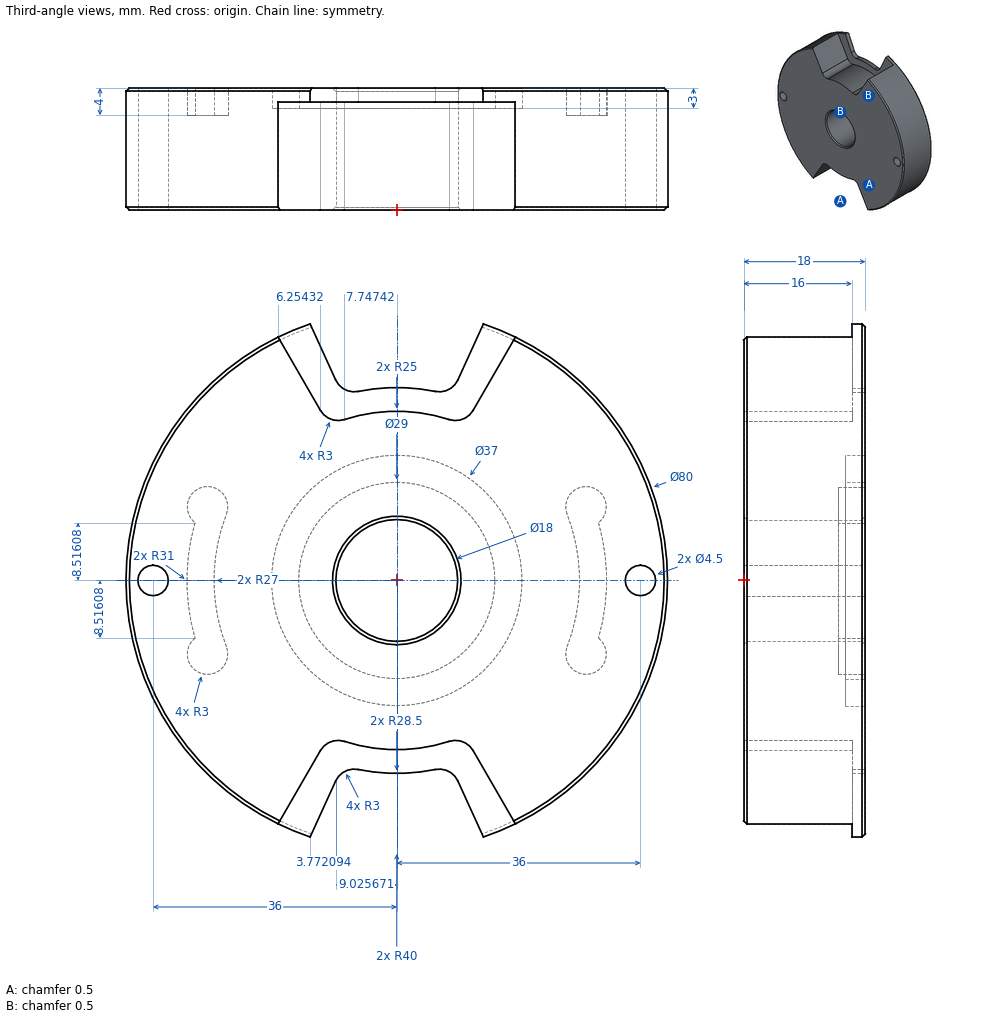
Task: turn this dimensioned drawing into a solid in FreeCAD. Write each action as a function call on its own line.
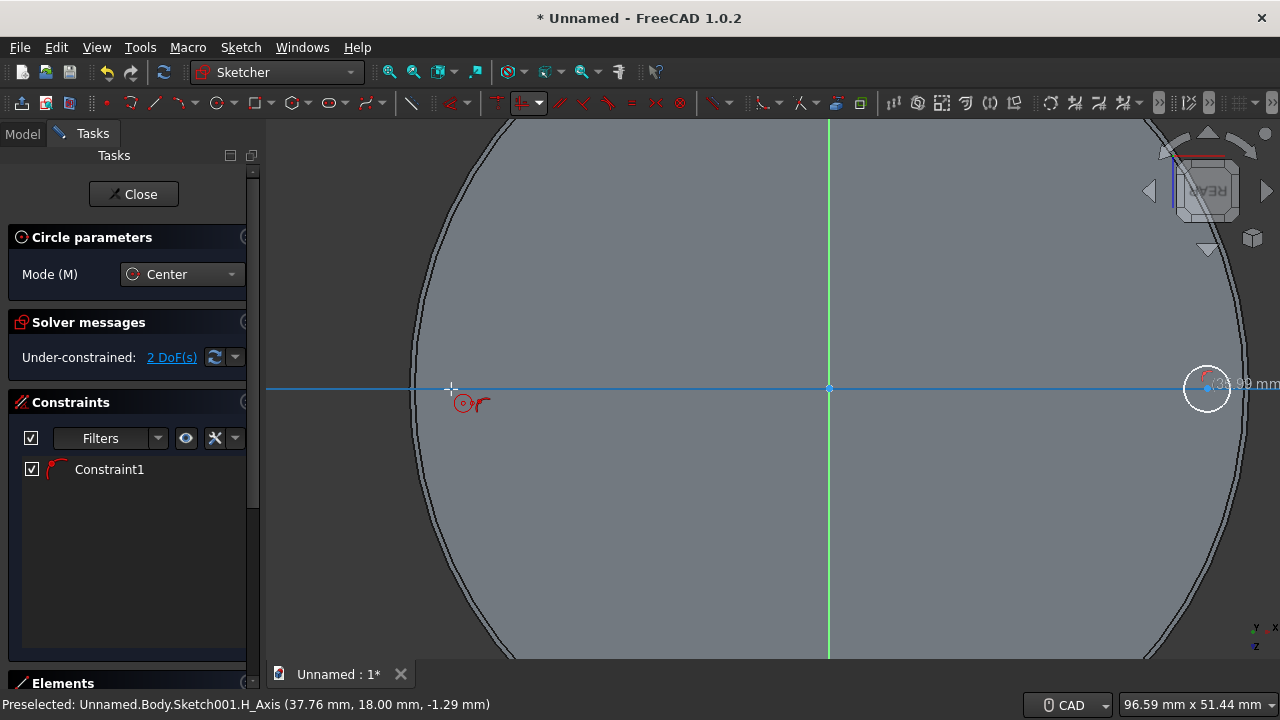
click(451, 389)
click(468, 372)
key(Escape)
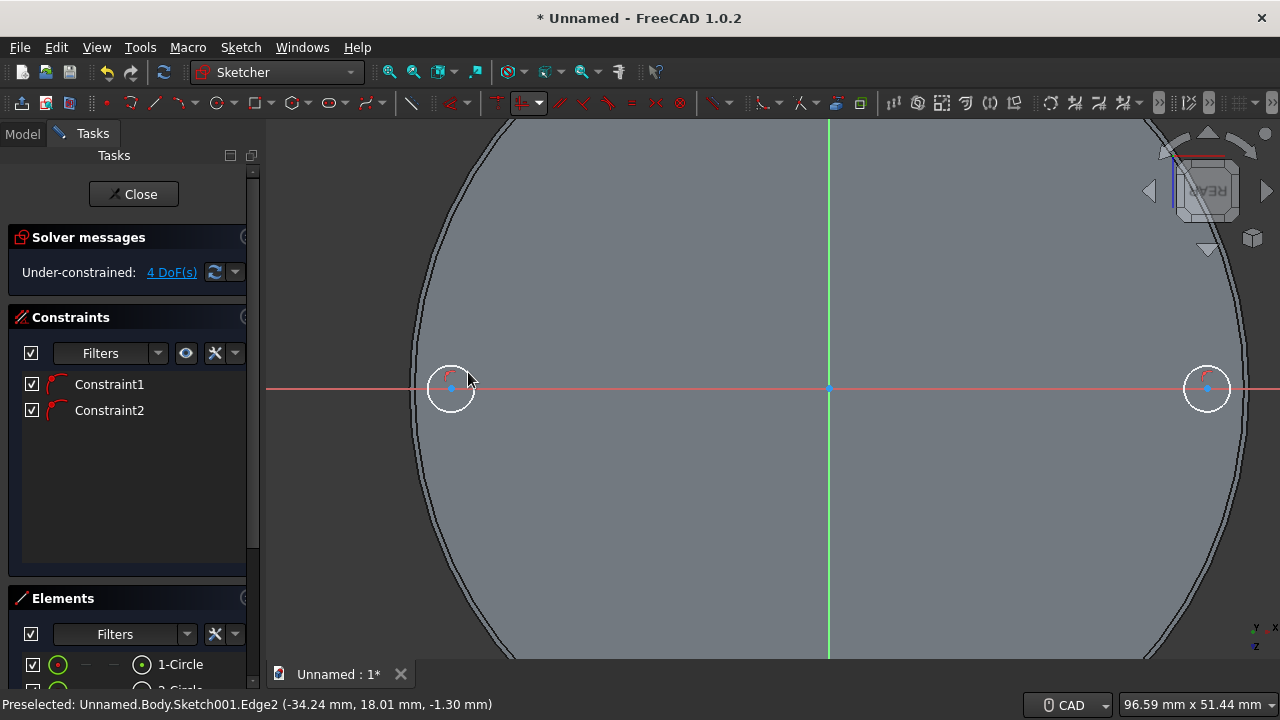
scroll(451, 389, down, 2)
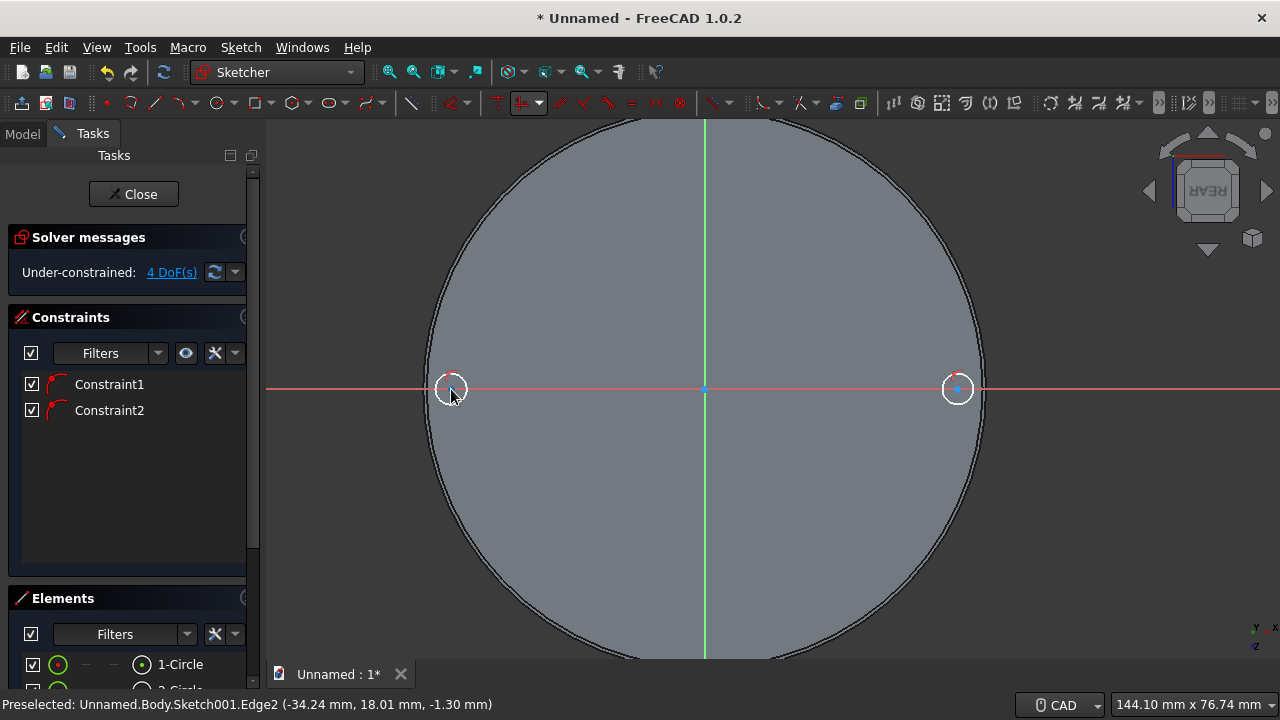
scroll(969, 378, up, 2)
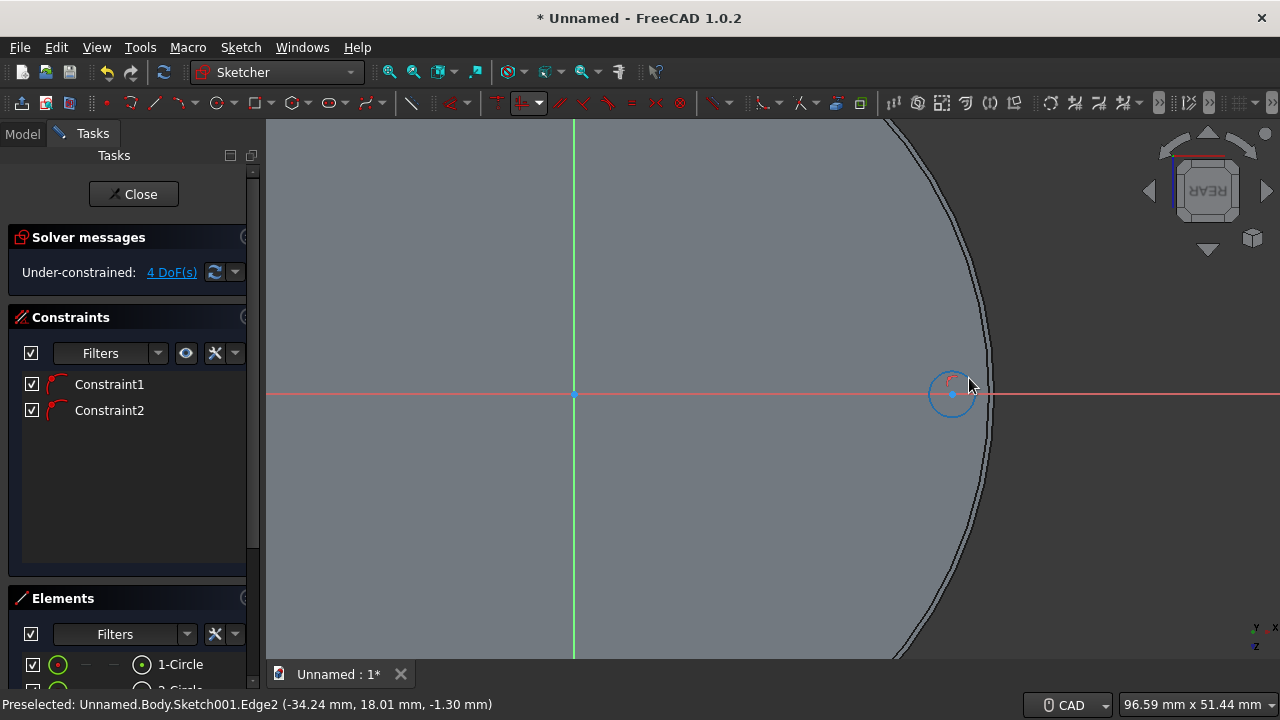
click(968, 378)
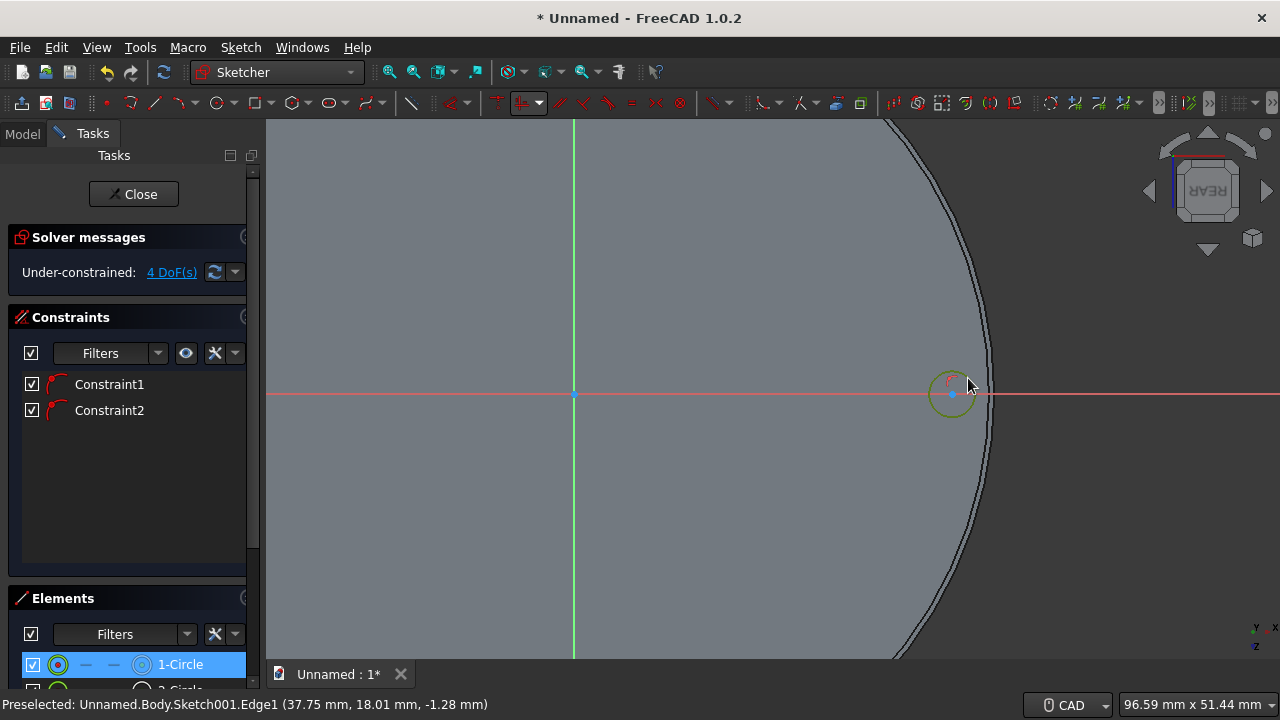
scroll(969, 378, down, 2)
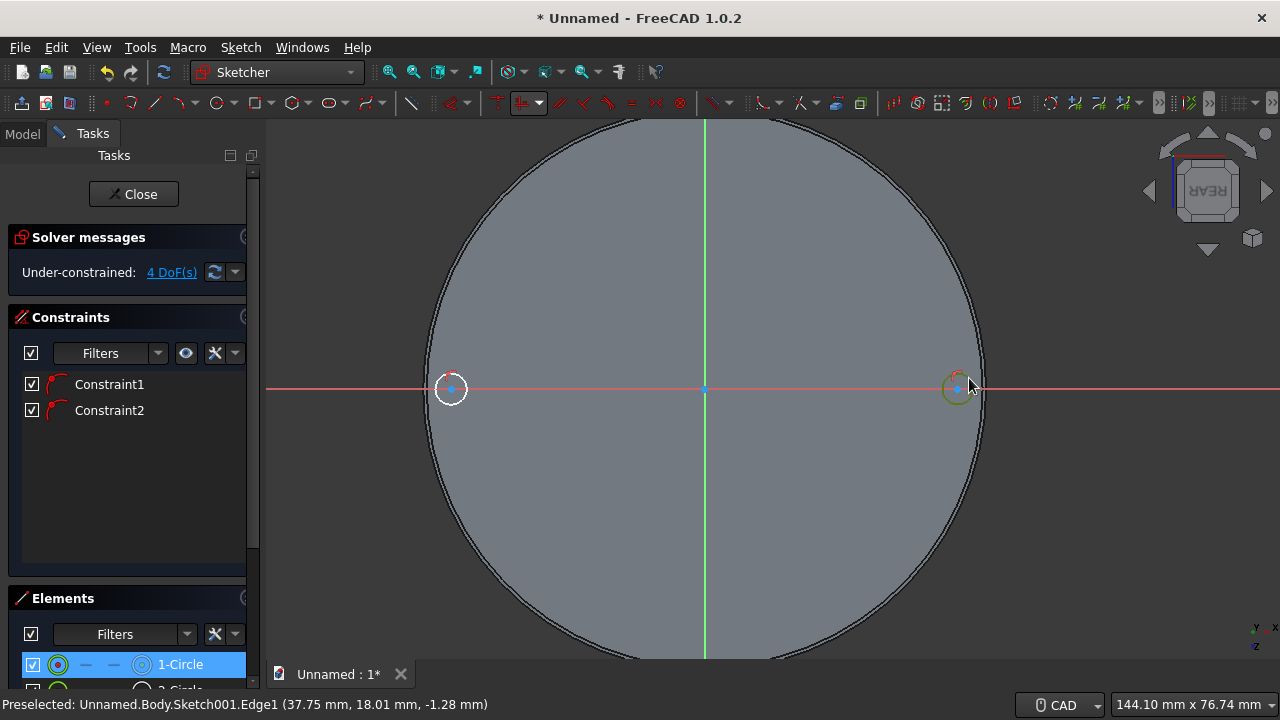
scroll(462, 378, up, 2)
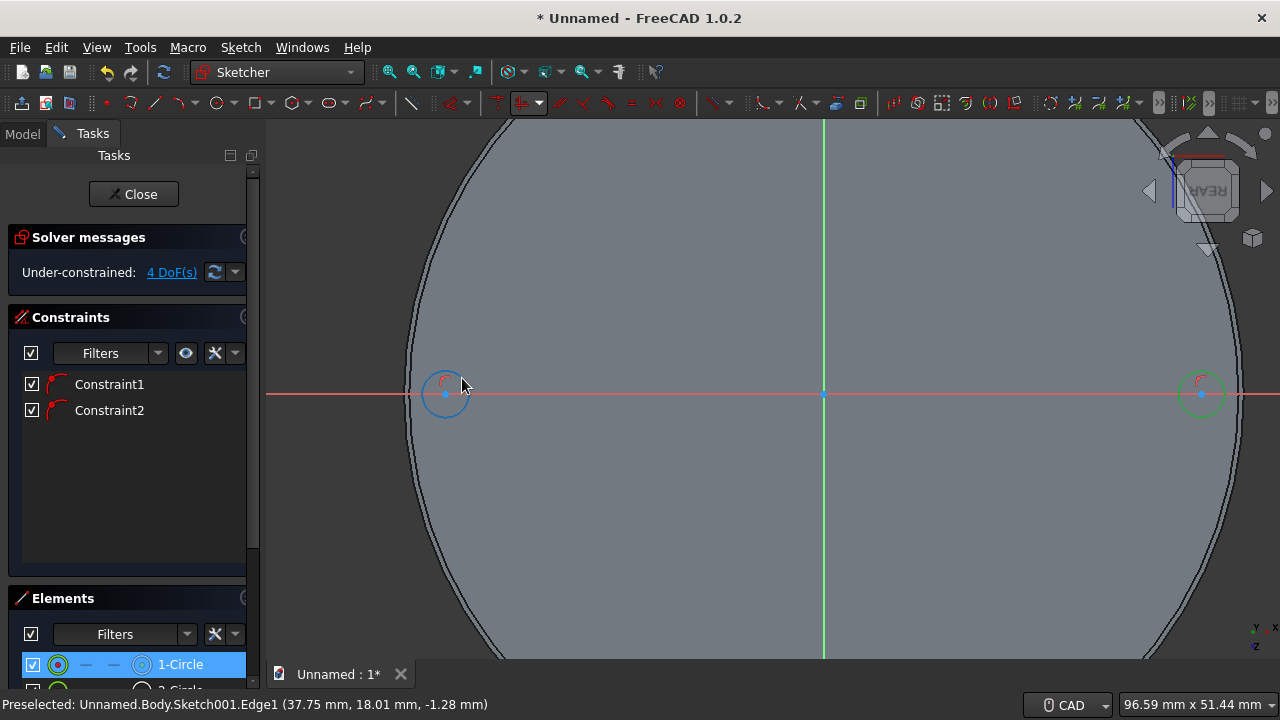
click(462, 378)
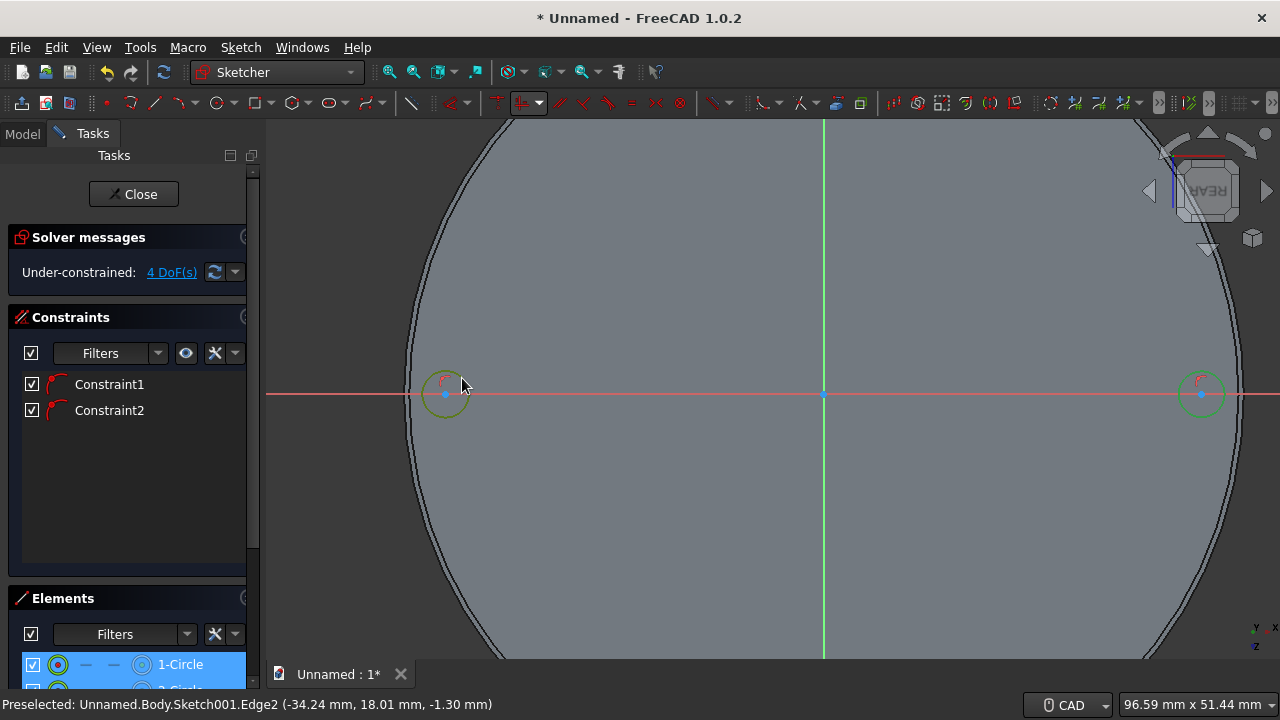
click(632, 104)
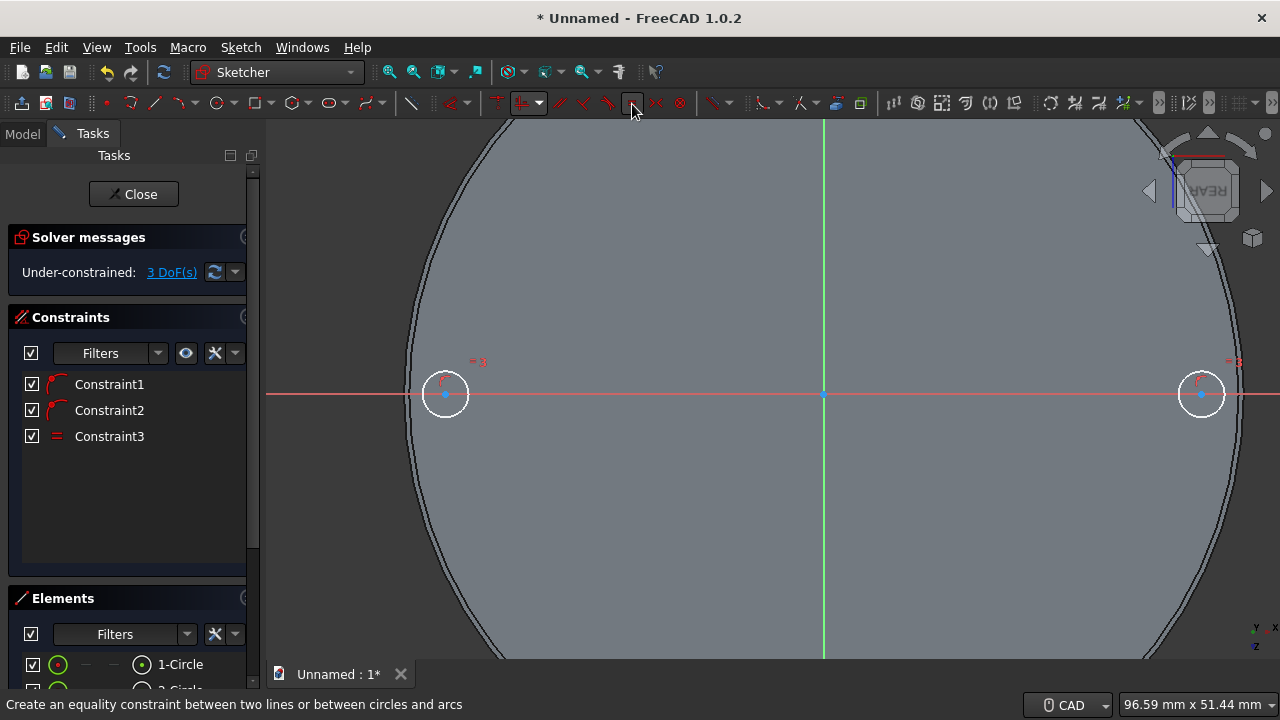
click(450, 104)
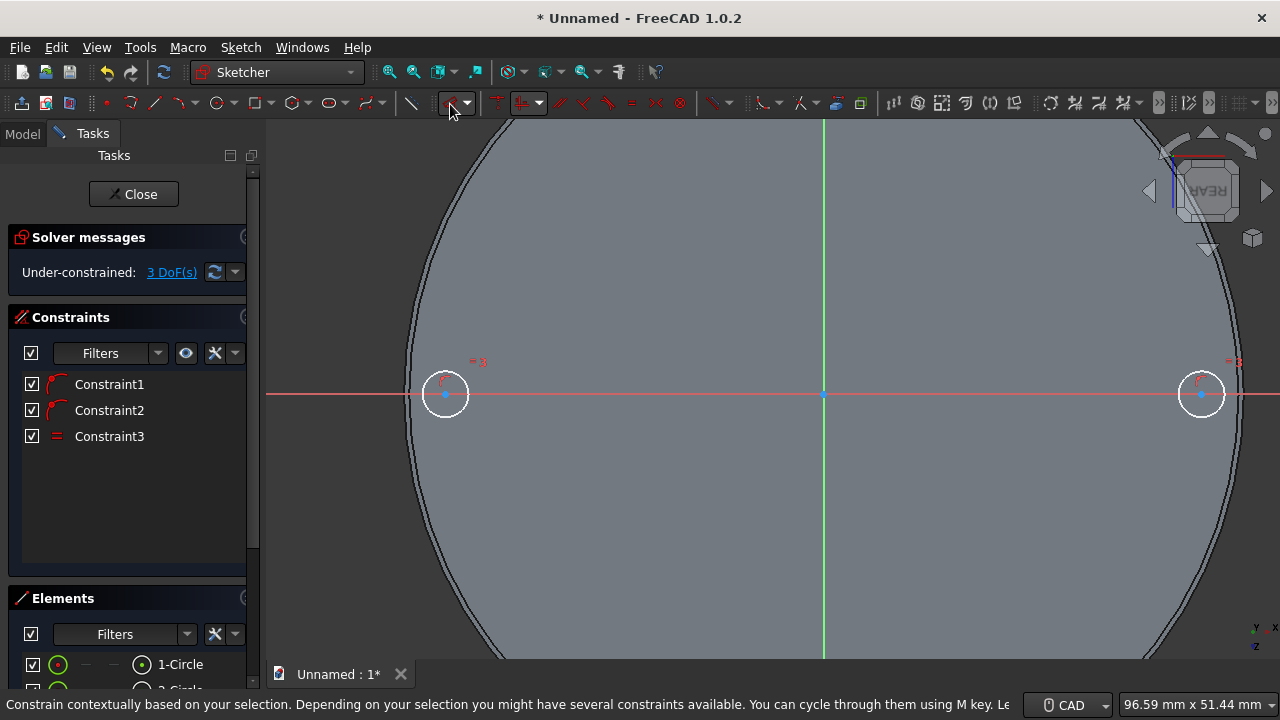
scroll(462, 378, down, 2)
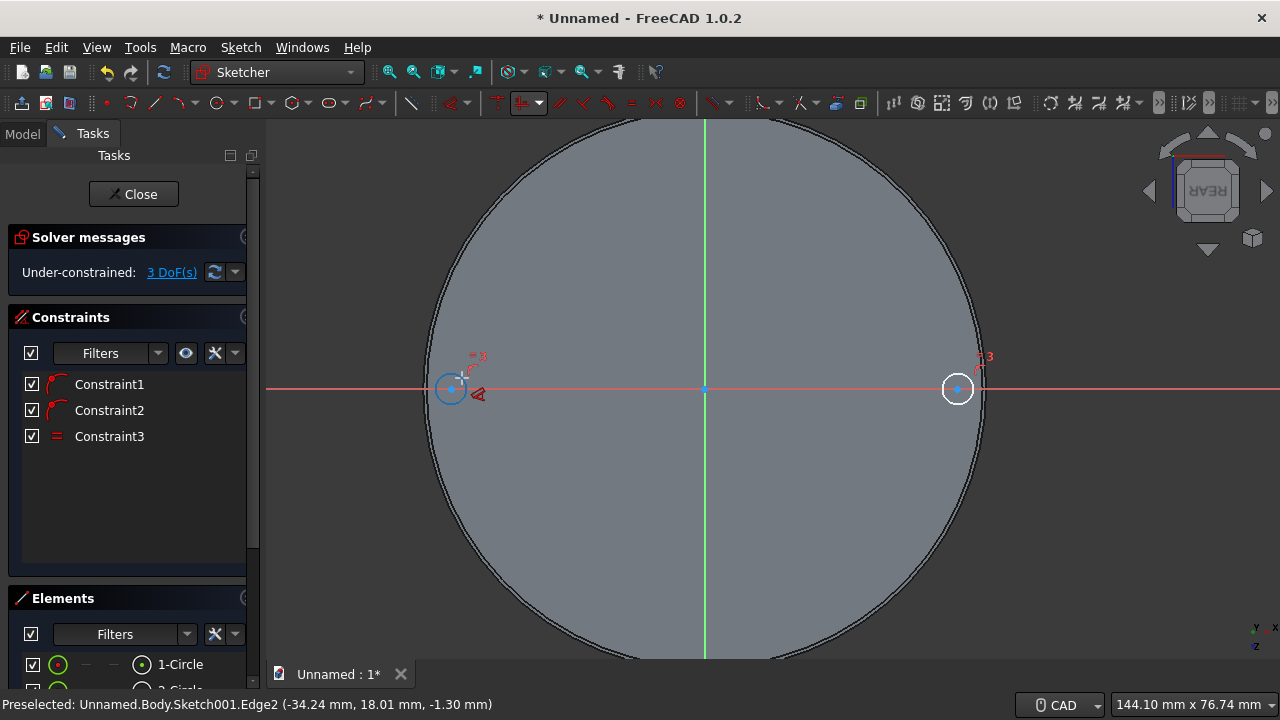
scroll(969, 378, up, 2)